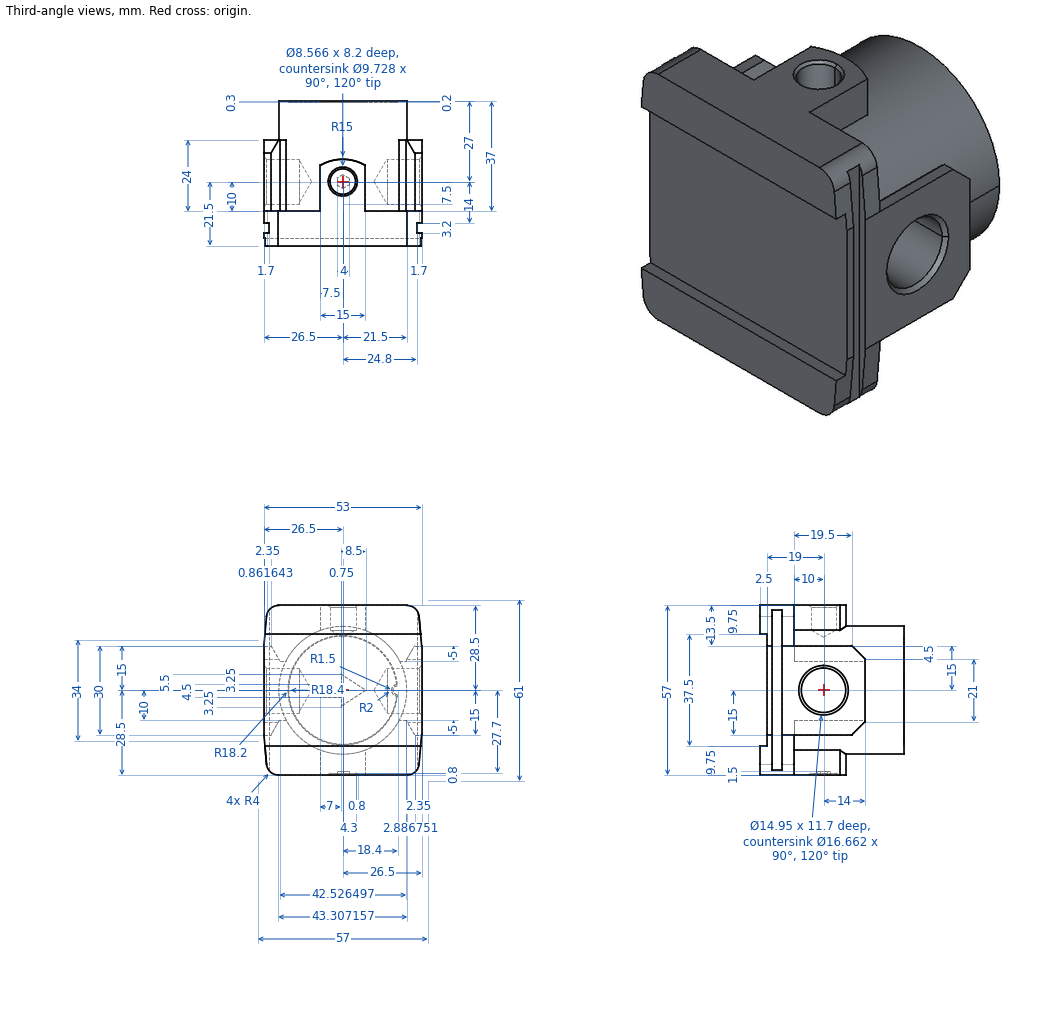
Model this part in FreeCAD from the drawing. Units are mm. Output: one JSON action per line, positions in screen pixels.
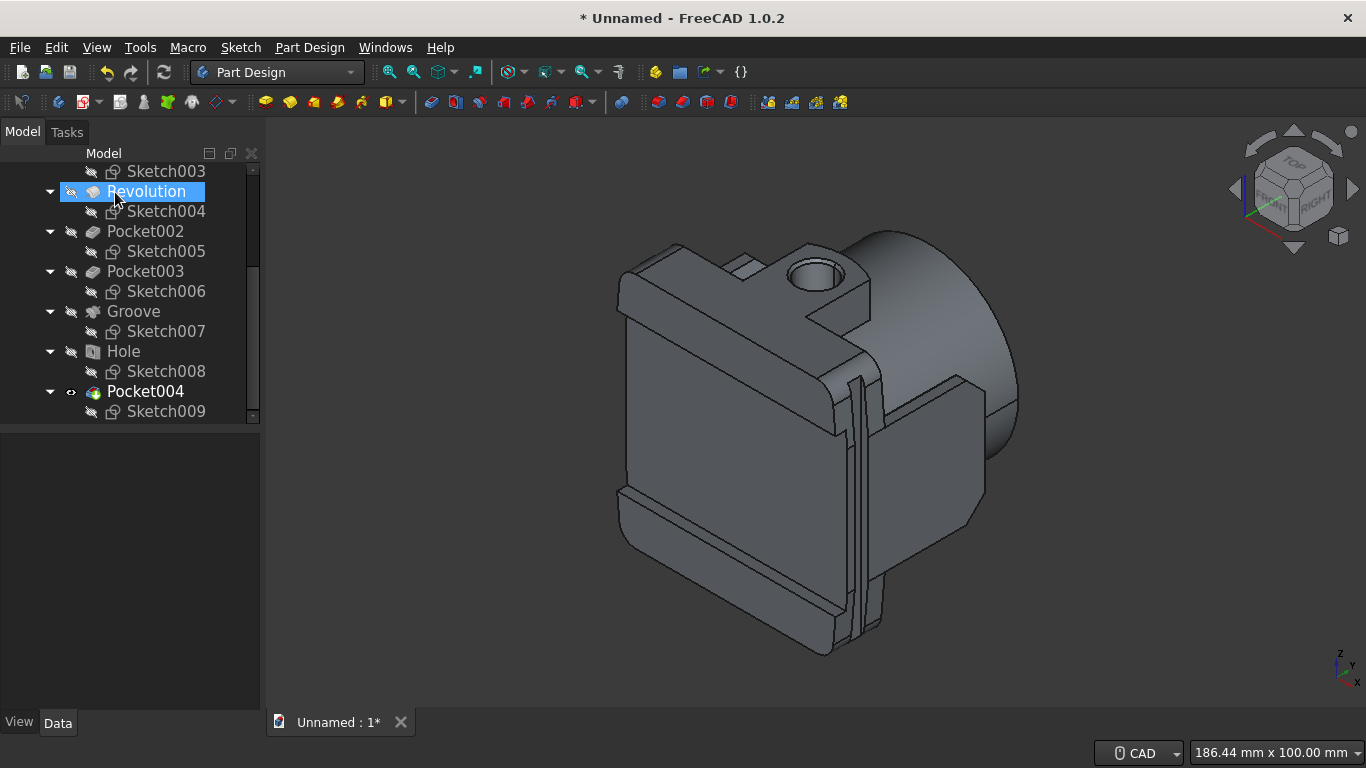
{"action": "left_click", "coordinate": [927, 475]}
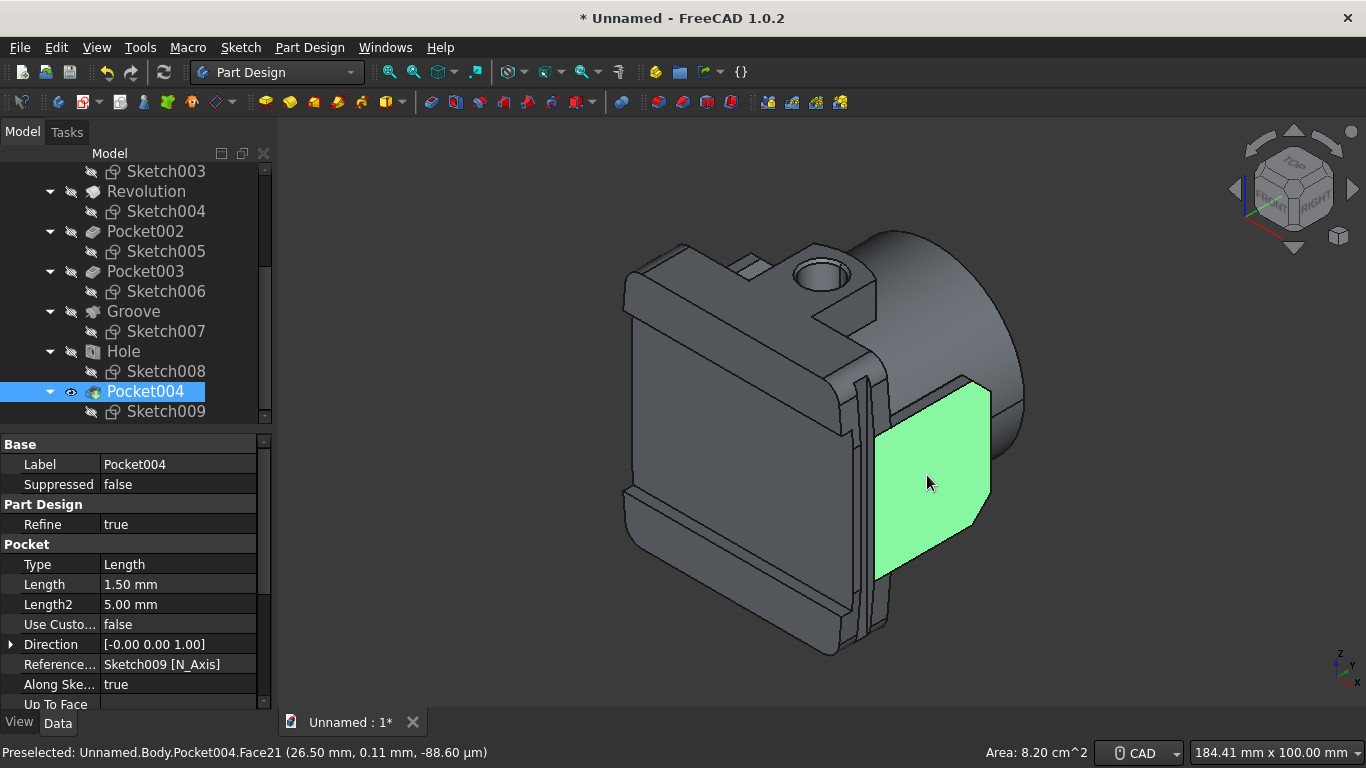
{"action": "left_click", "coordinate": [84, 102]}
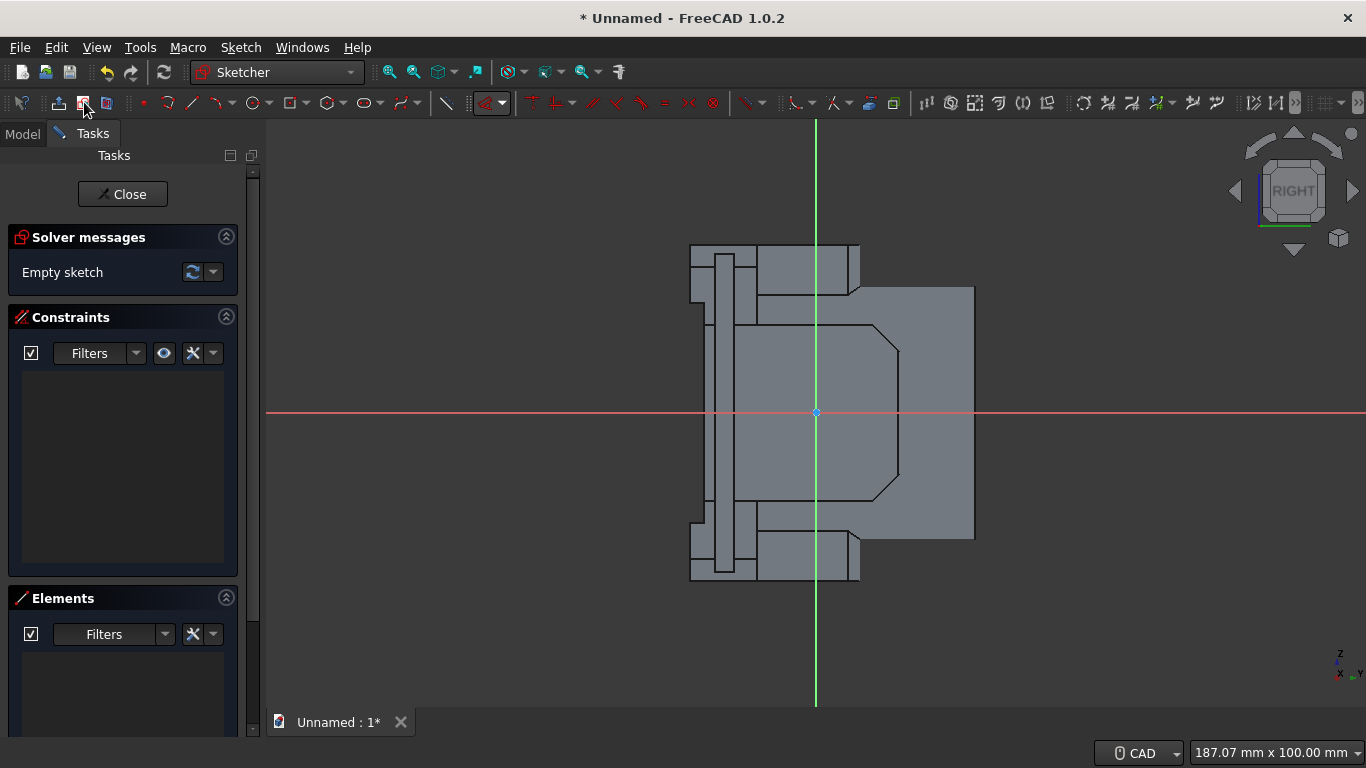
{"action": "scroll", "coordinate": [838, 413], "scroll_direction": "up", "scroll_amount": 7}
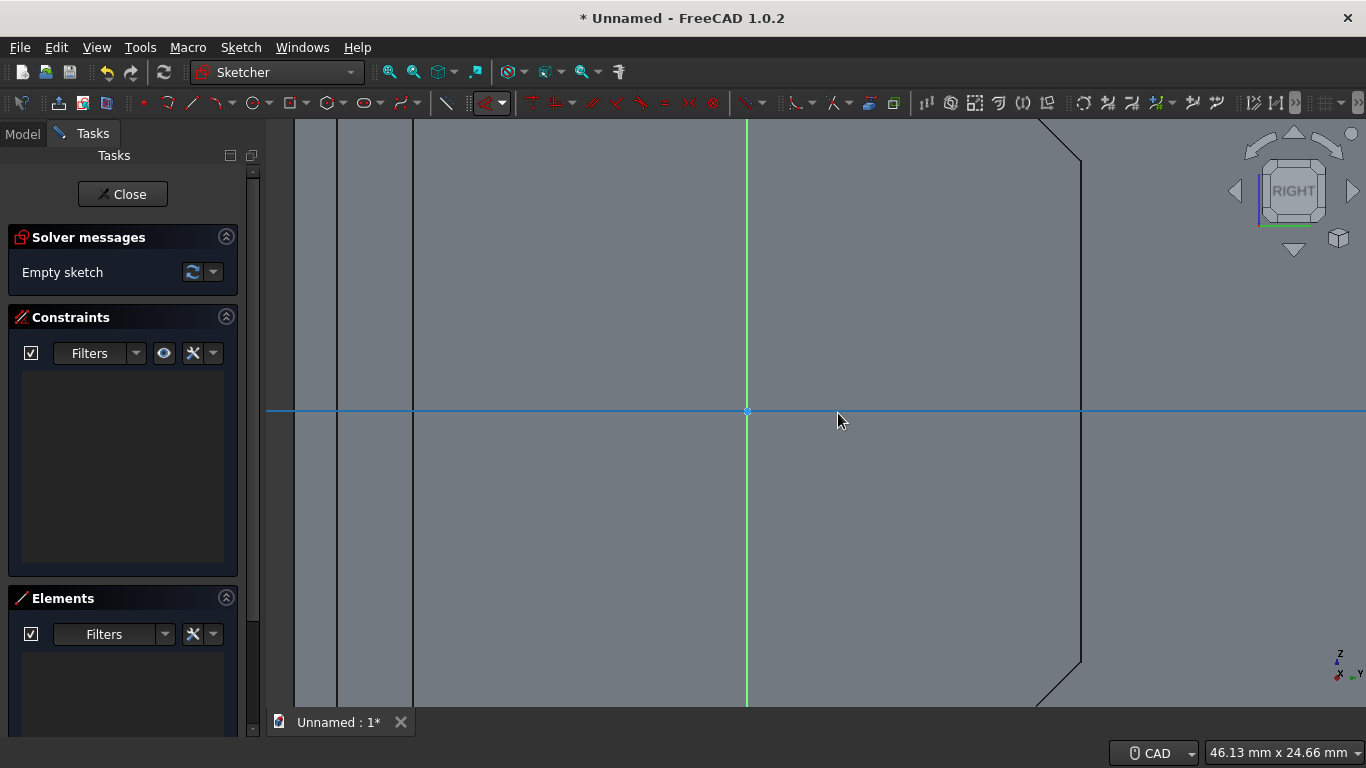
{"action": "left_click", "coordinate": [254, 104]}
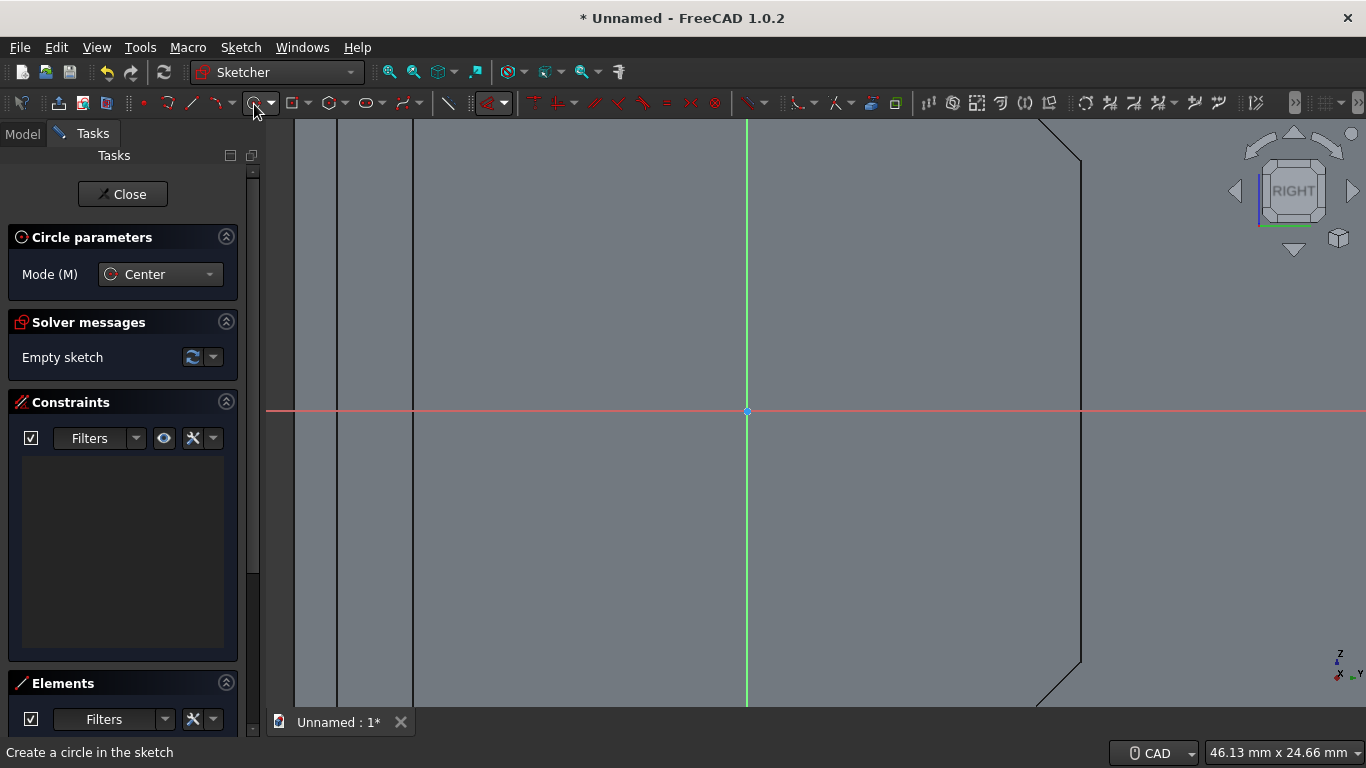
{"action": "left_click", "coordinate": [747, 411]}
{"action": "mouse_move", "coordinate": [873, 285]}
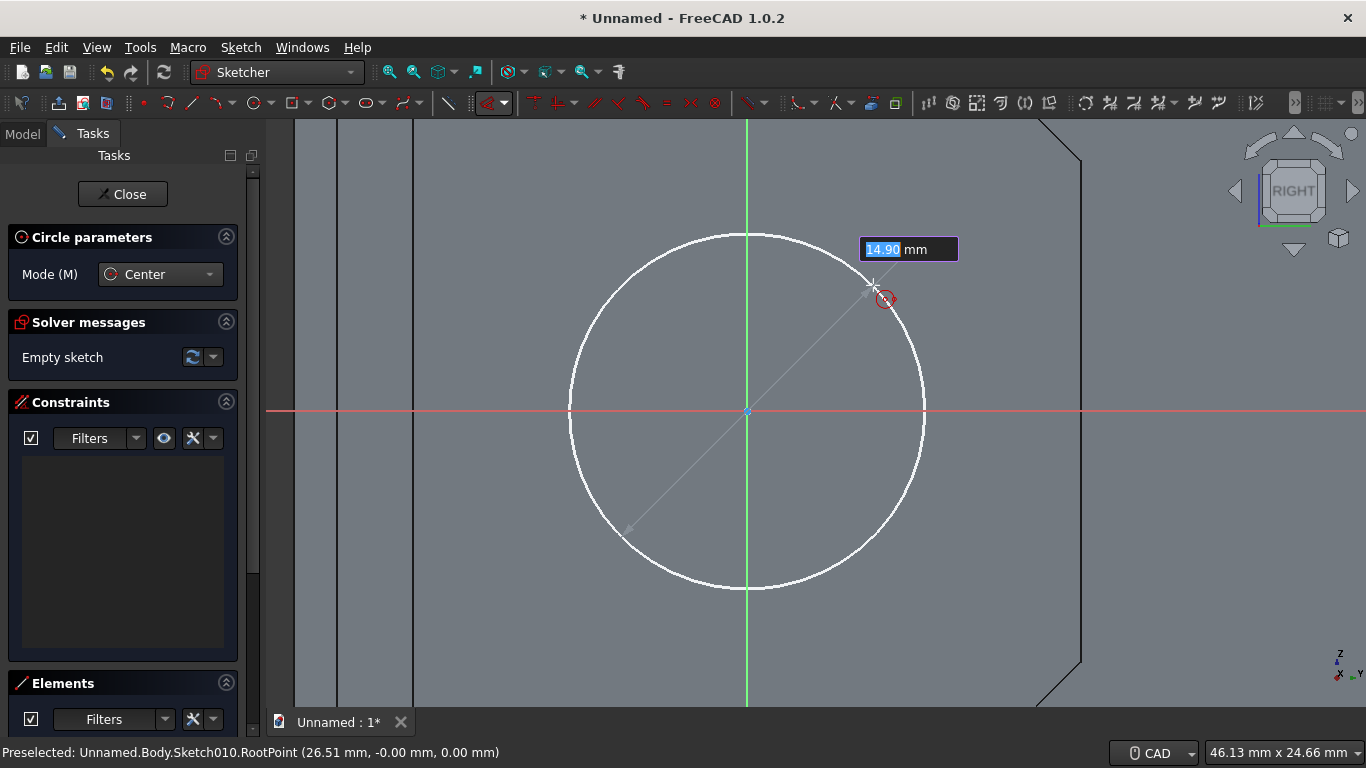
{"action": "type", "text": "14.95"}
{"action": "key", "text": "Return"}
{"action": "key", "text": "Escape"}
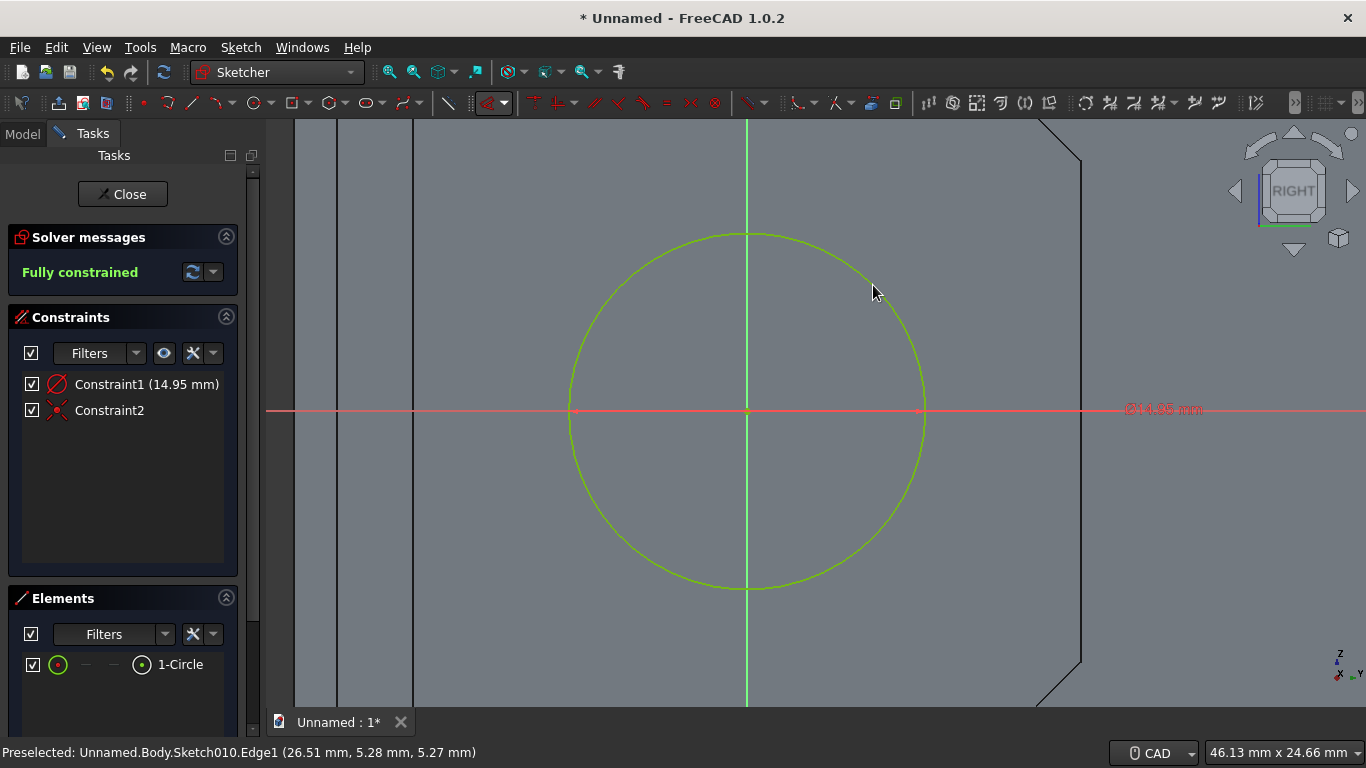
{"action": "left_click", "coordinate": [123, 194]}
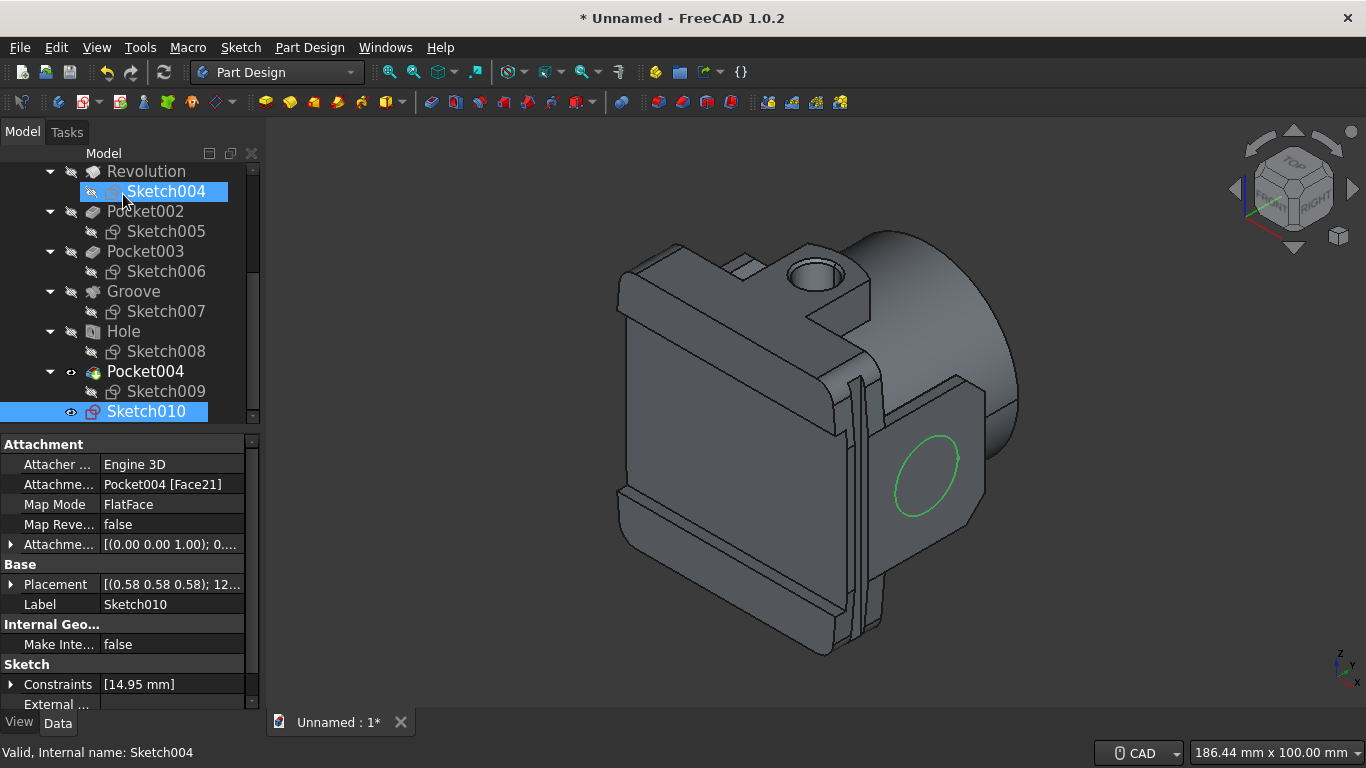
{"action": "left_click", "coordinate": [456, 102]}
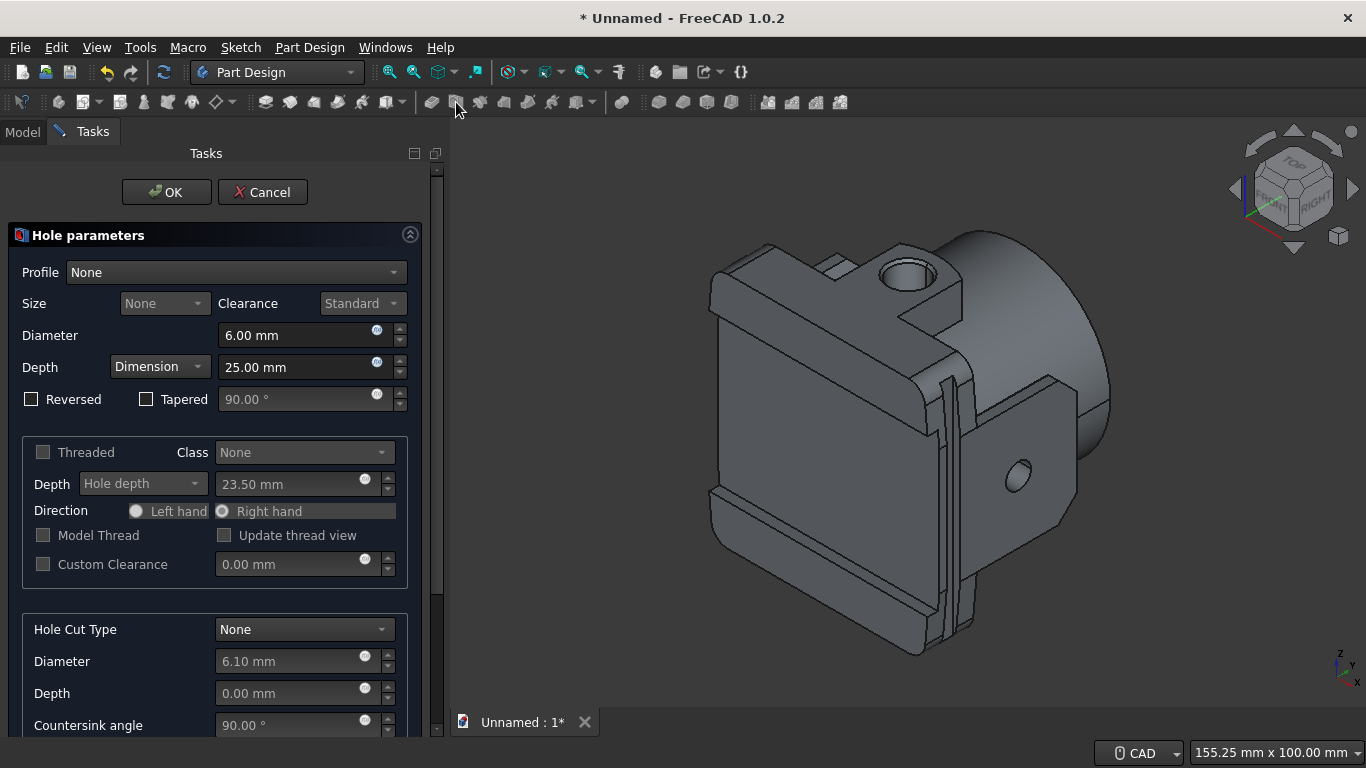
{"action": "triple_click", "coordinate": [305, 335]}